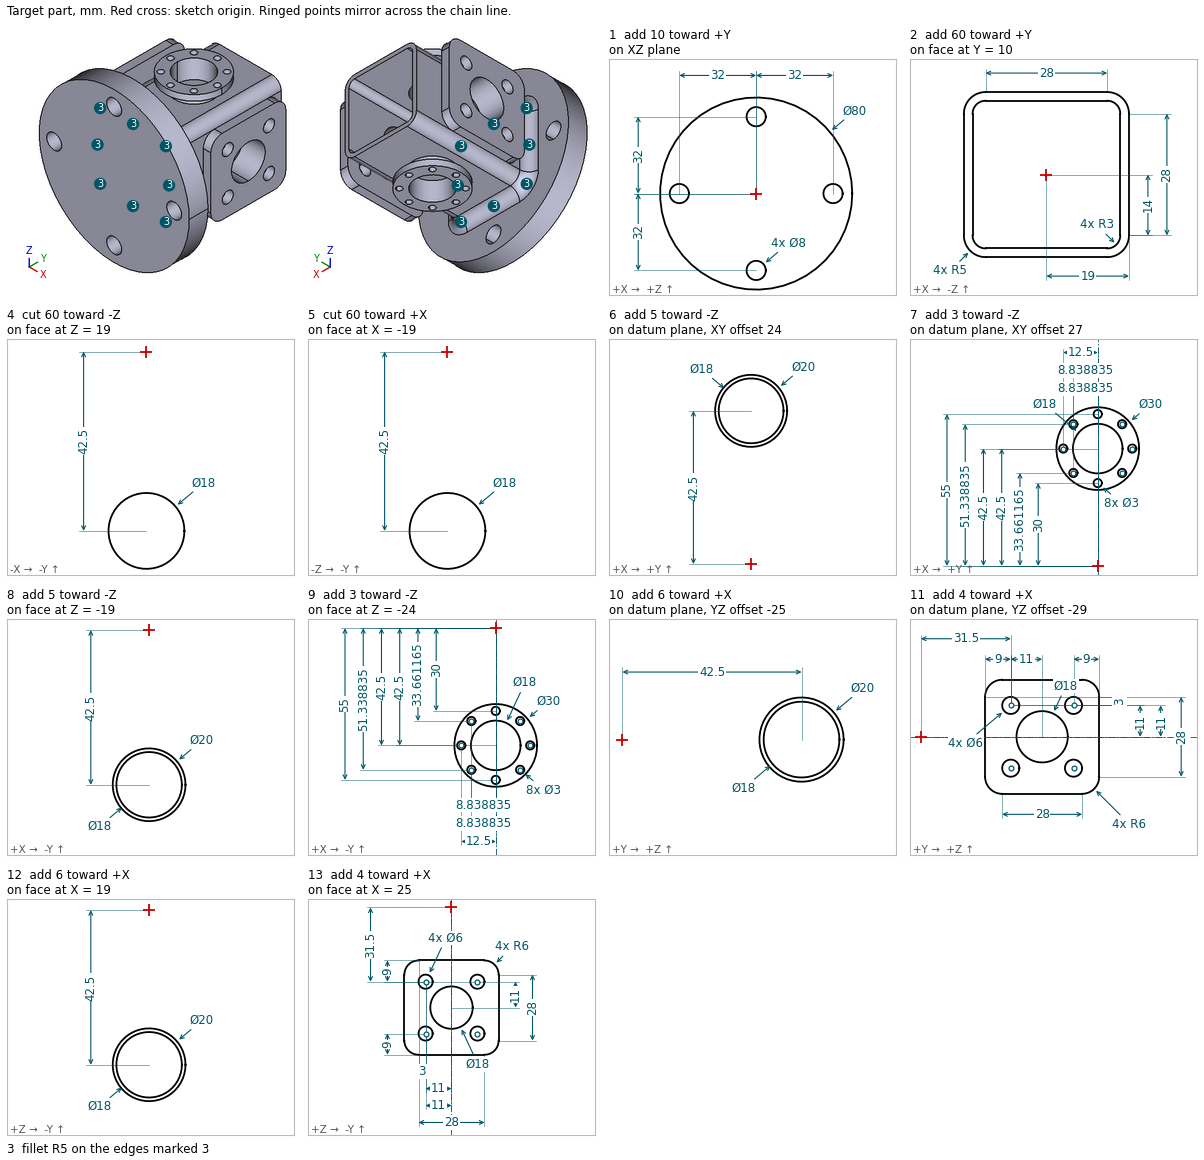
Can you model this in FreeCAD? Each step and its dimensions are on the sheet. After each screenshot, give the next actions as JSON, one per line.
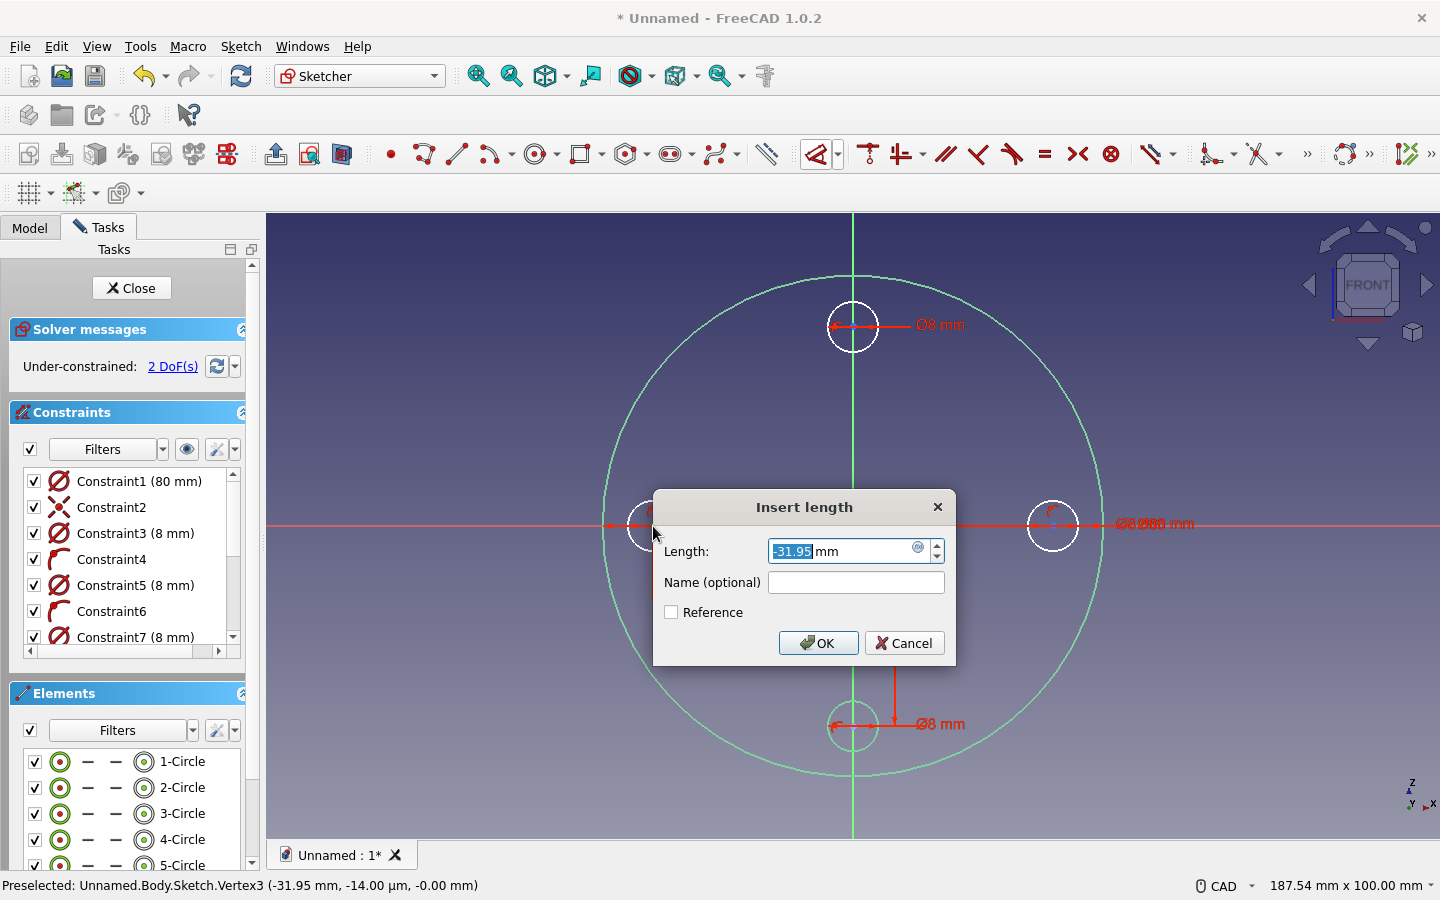
{"action": "type", "text": "-32"}
{"action": "key", "text": "Return"}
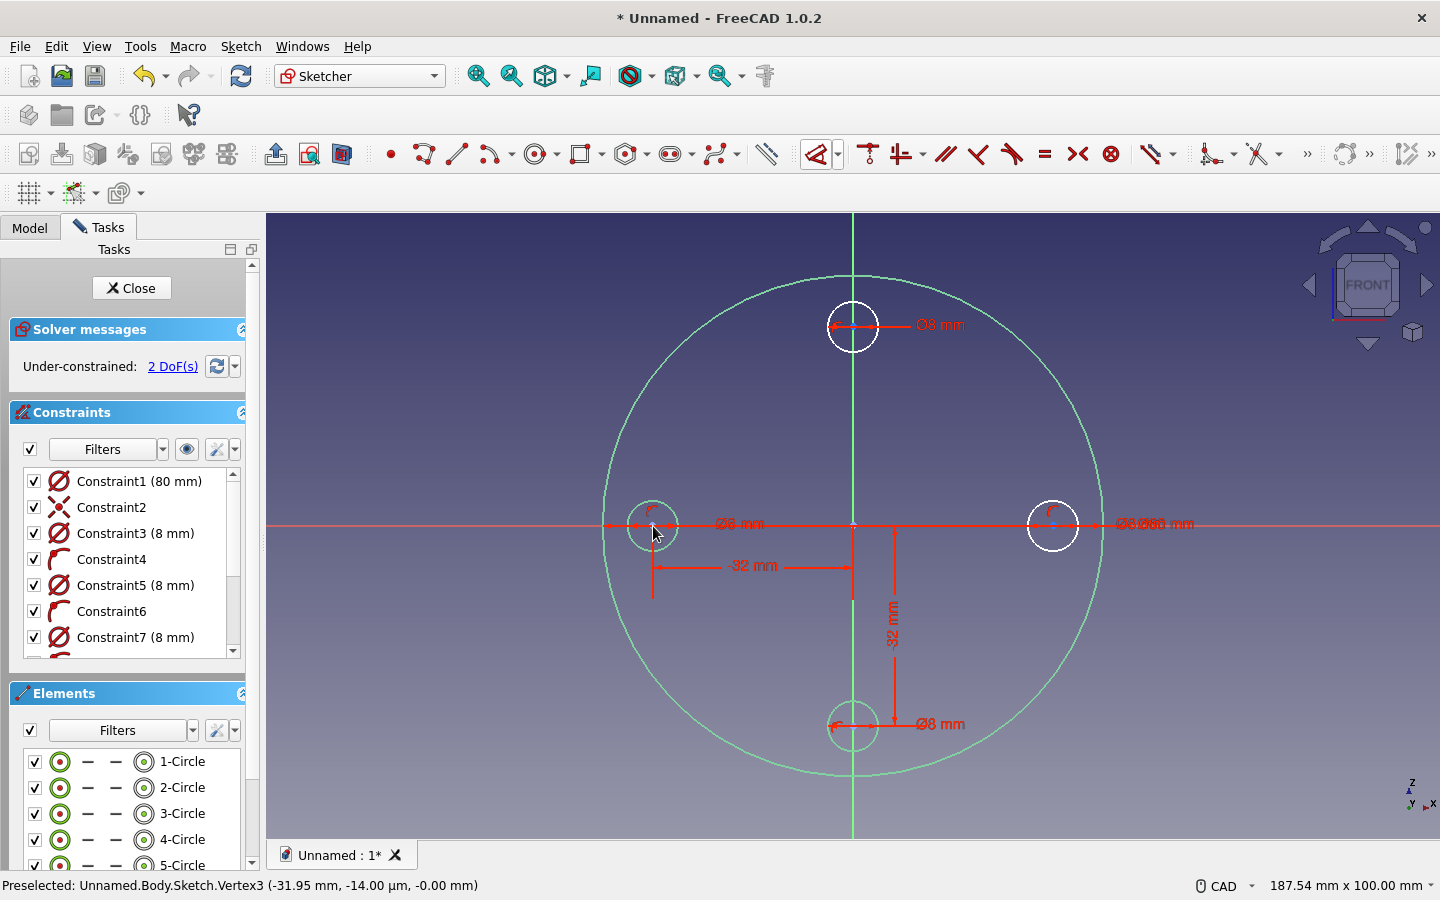
{"action": "left_click", "coordinate": [1053, 526]}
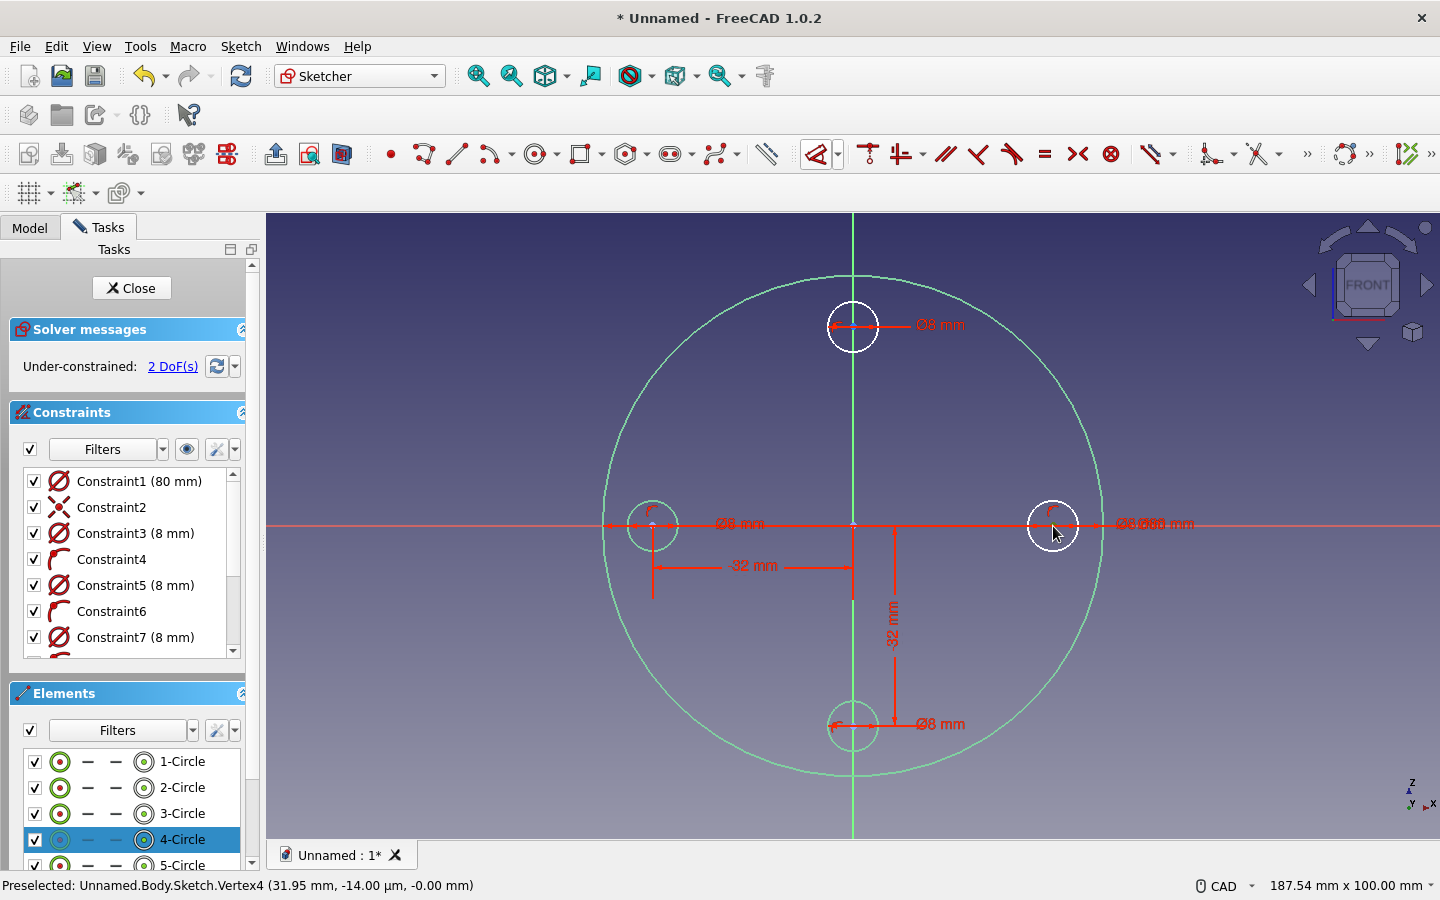
{"action": "left_click", "coordinate": [838, 154]}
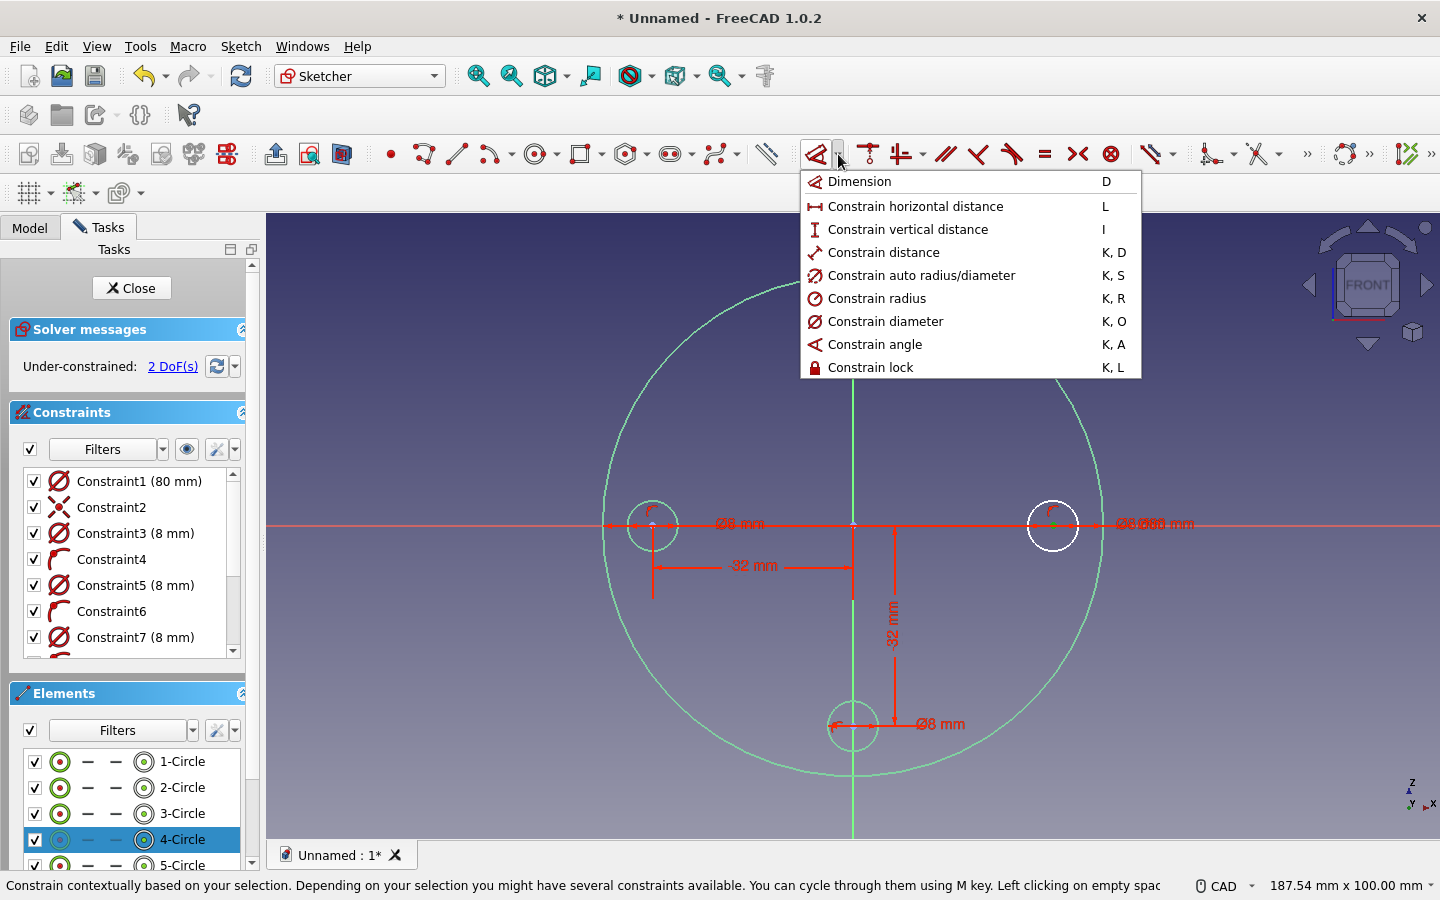
{"action": "left_click", "coordinate": [971, 206]}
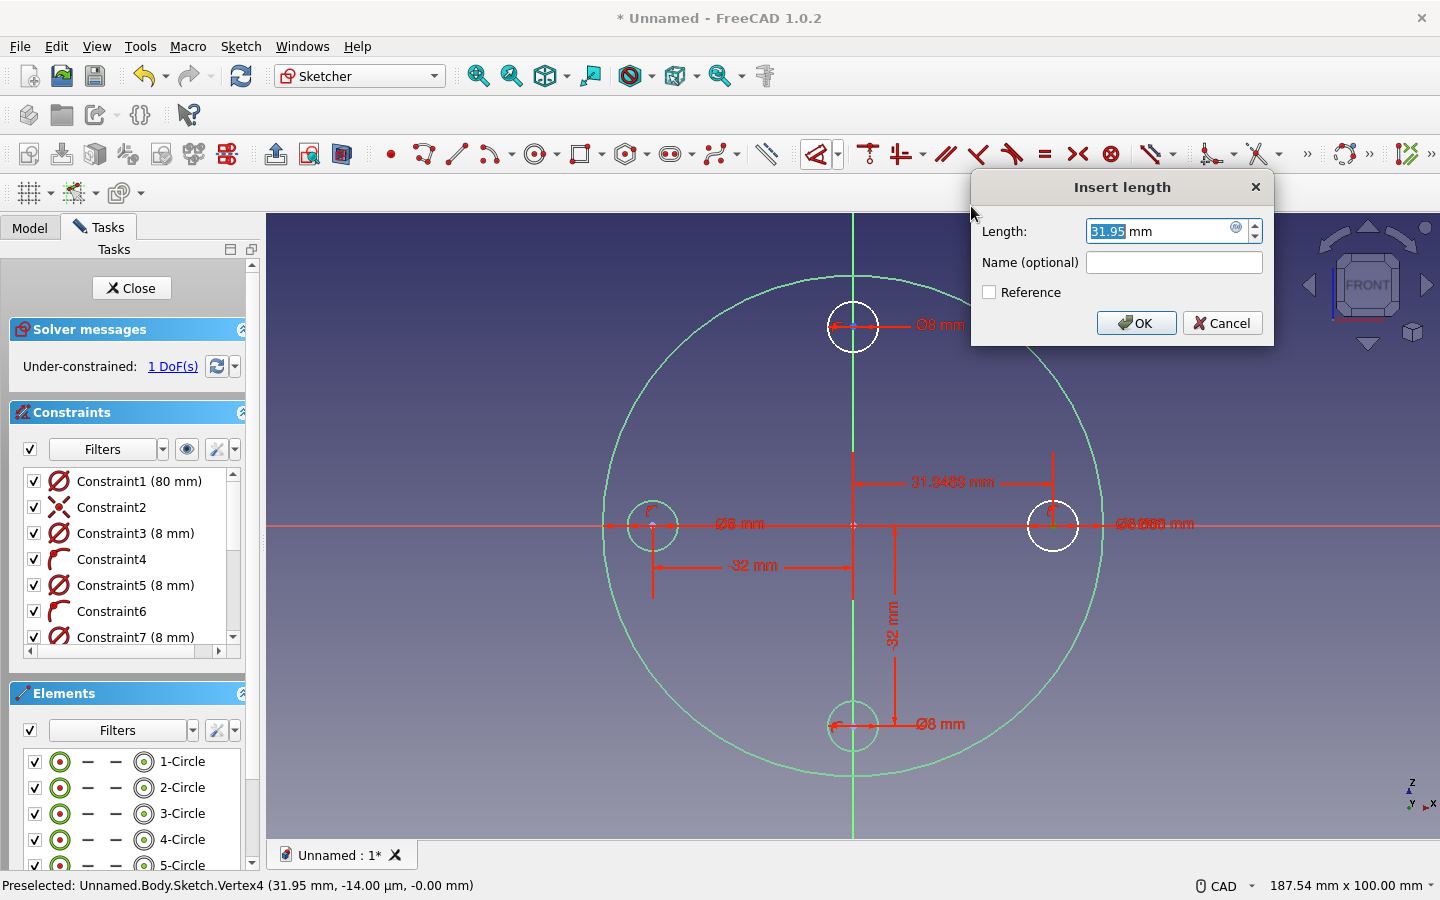
{"action": "type", "text": "32"}
{"action": "key", "text": "Return"}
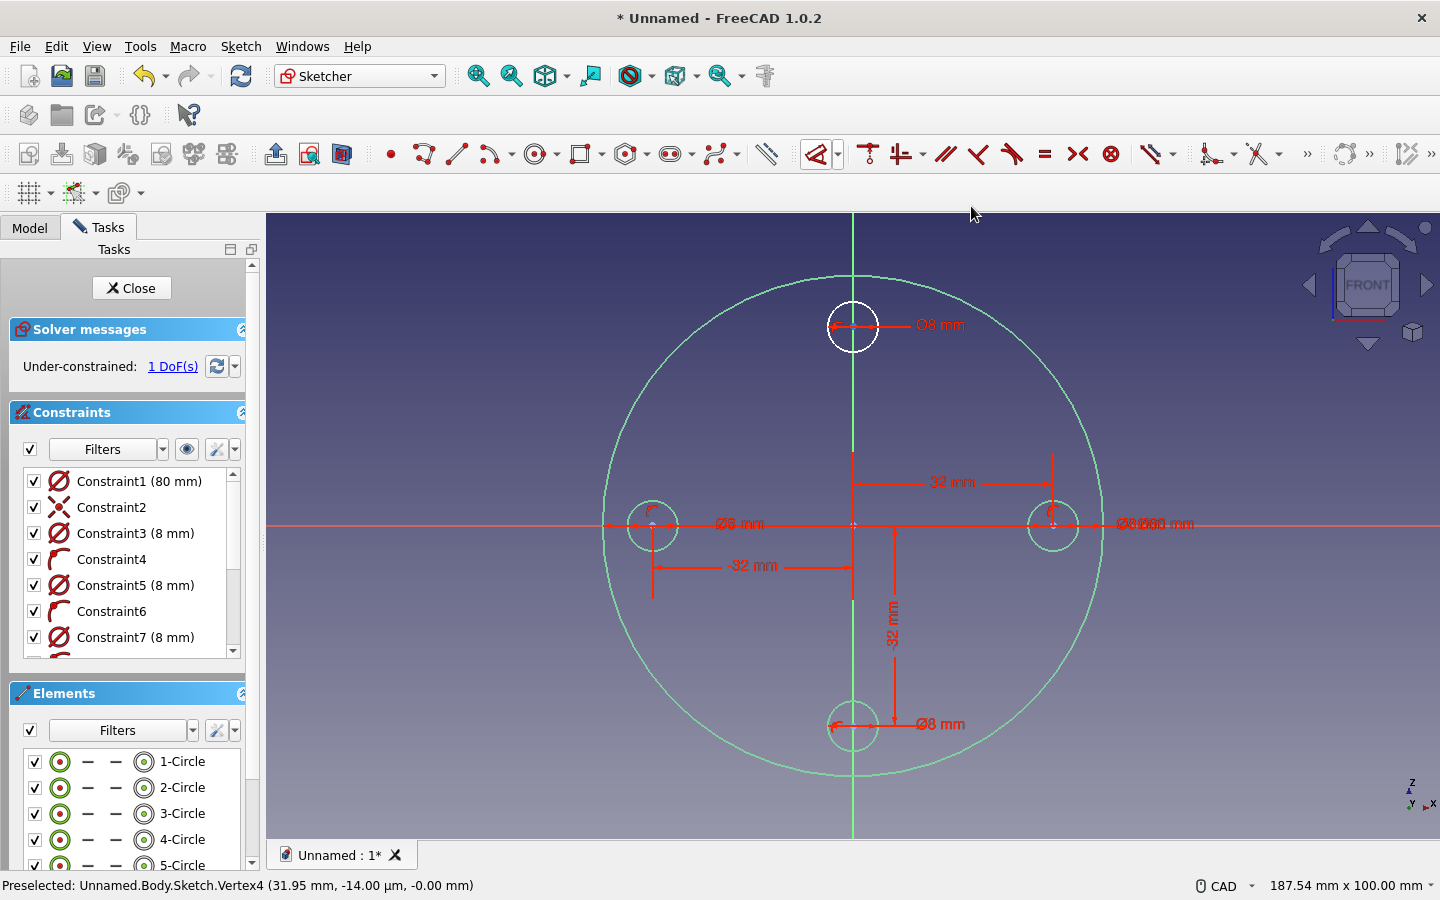
{"action": "left_click", "coordinate": [853, 327]}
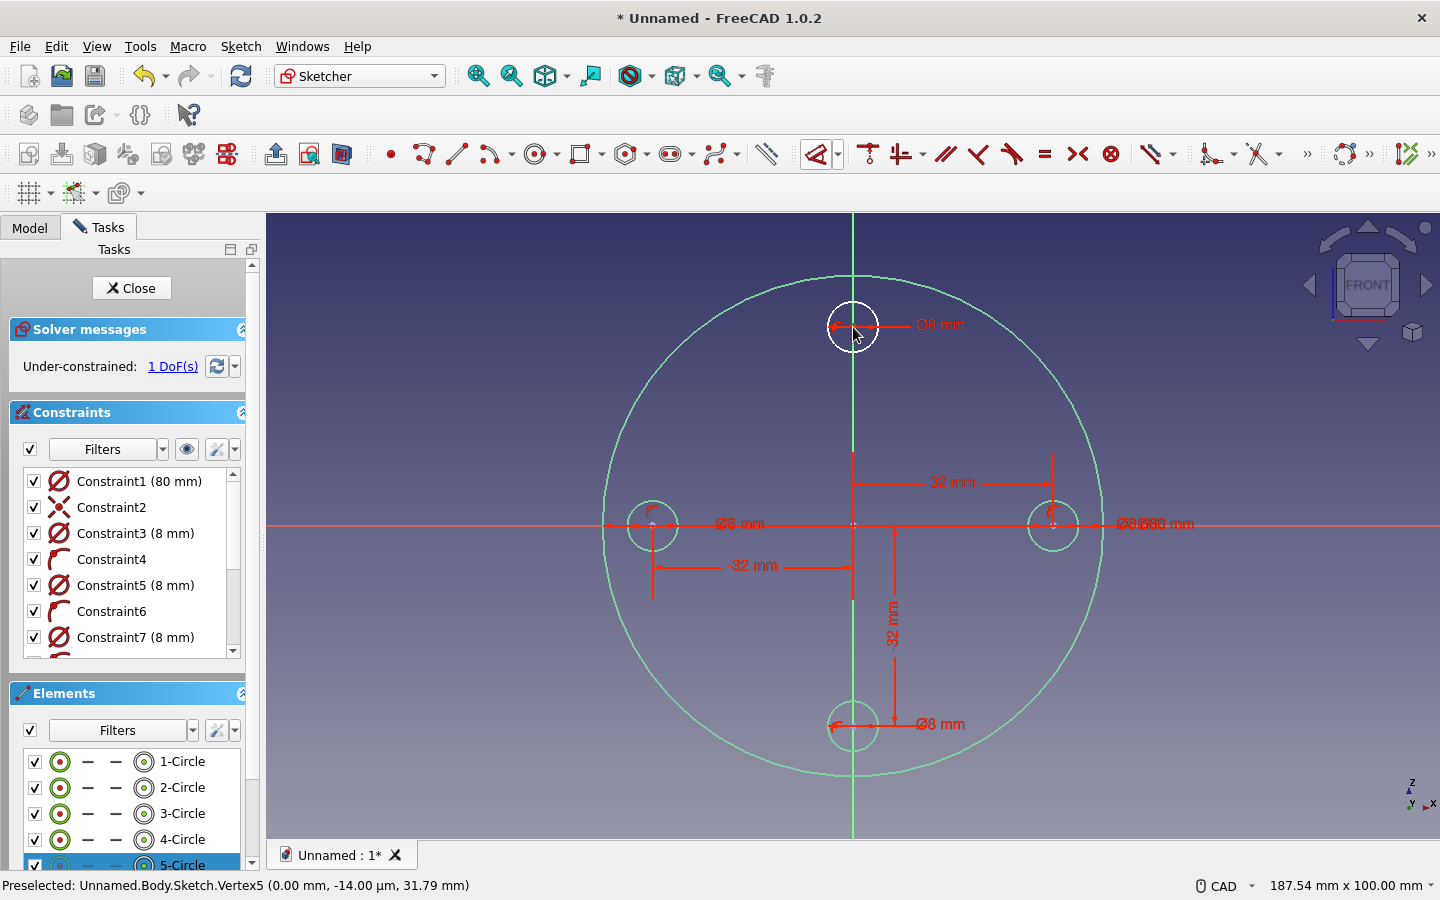
{"action": "key", "text": "i"}